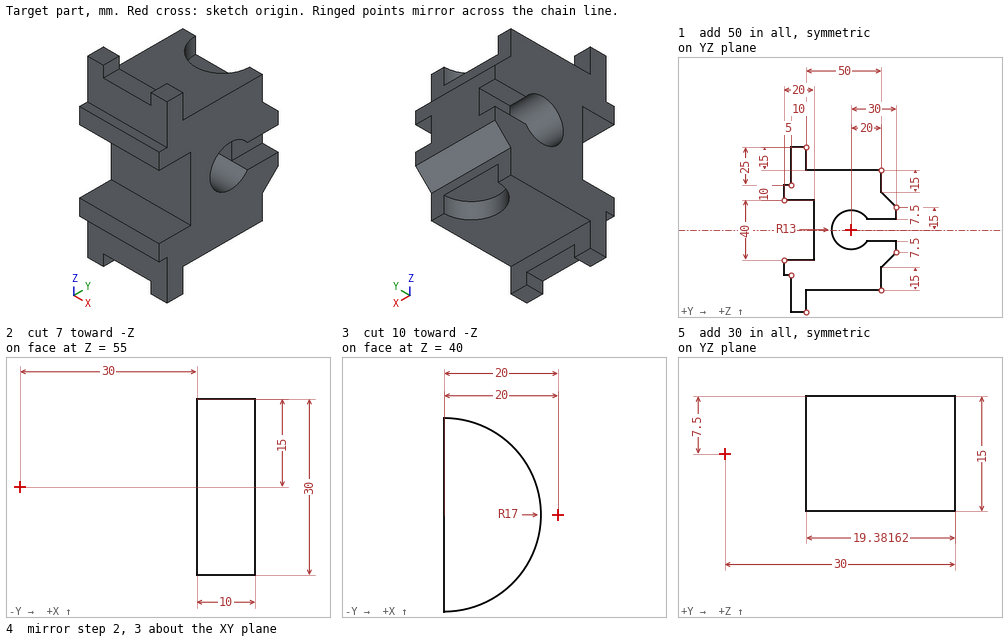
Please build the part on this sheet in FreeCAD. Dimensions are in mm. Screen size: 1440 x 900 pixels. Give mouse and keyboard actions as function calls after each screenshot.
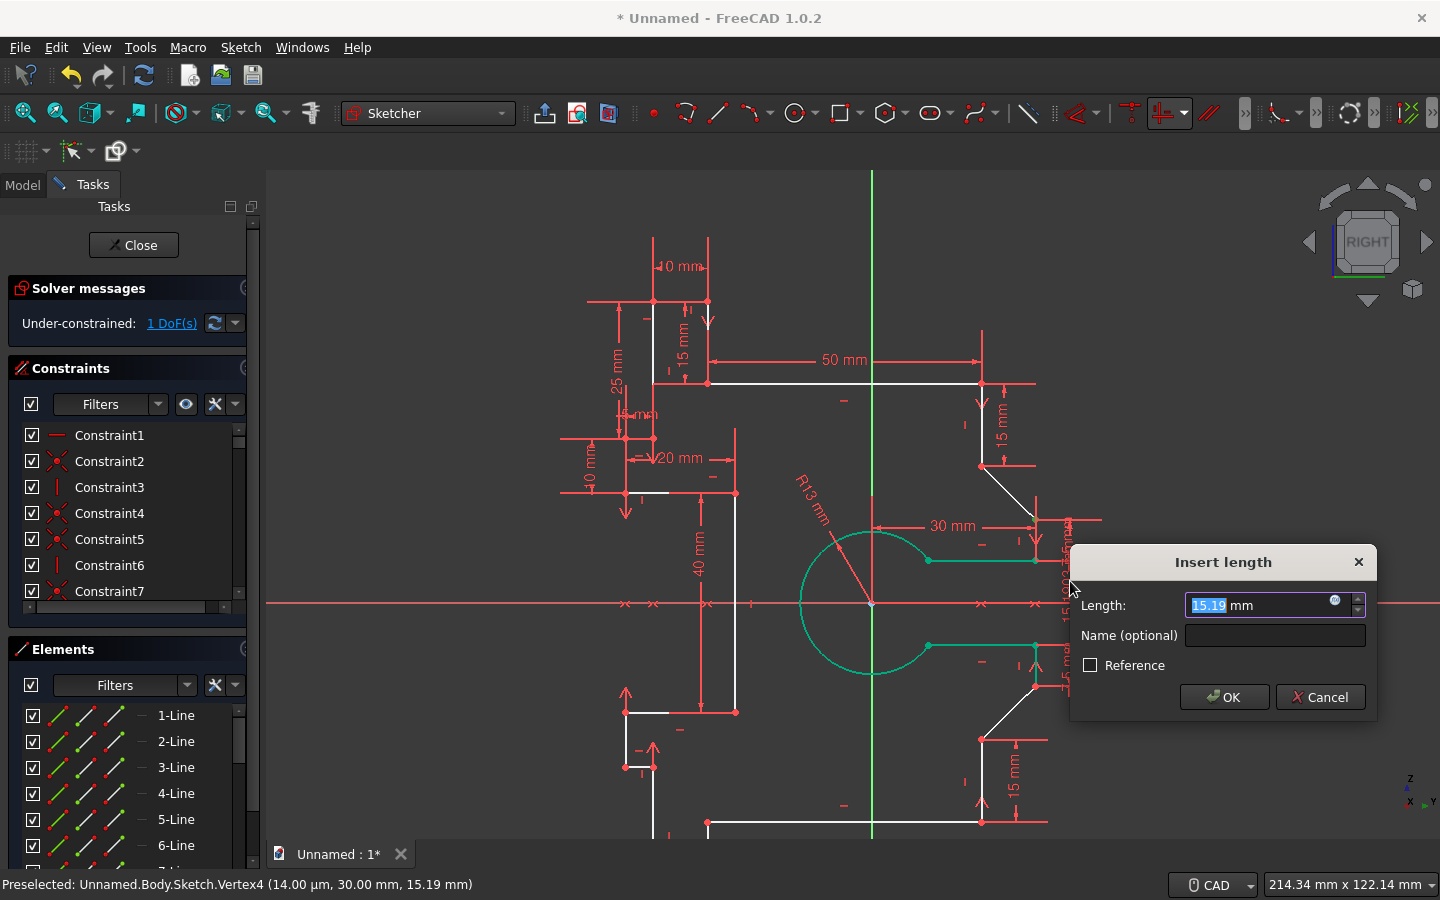
text(15)
key(Return)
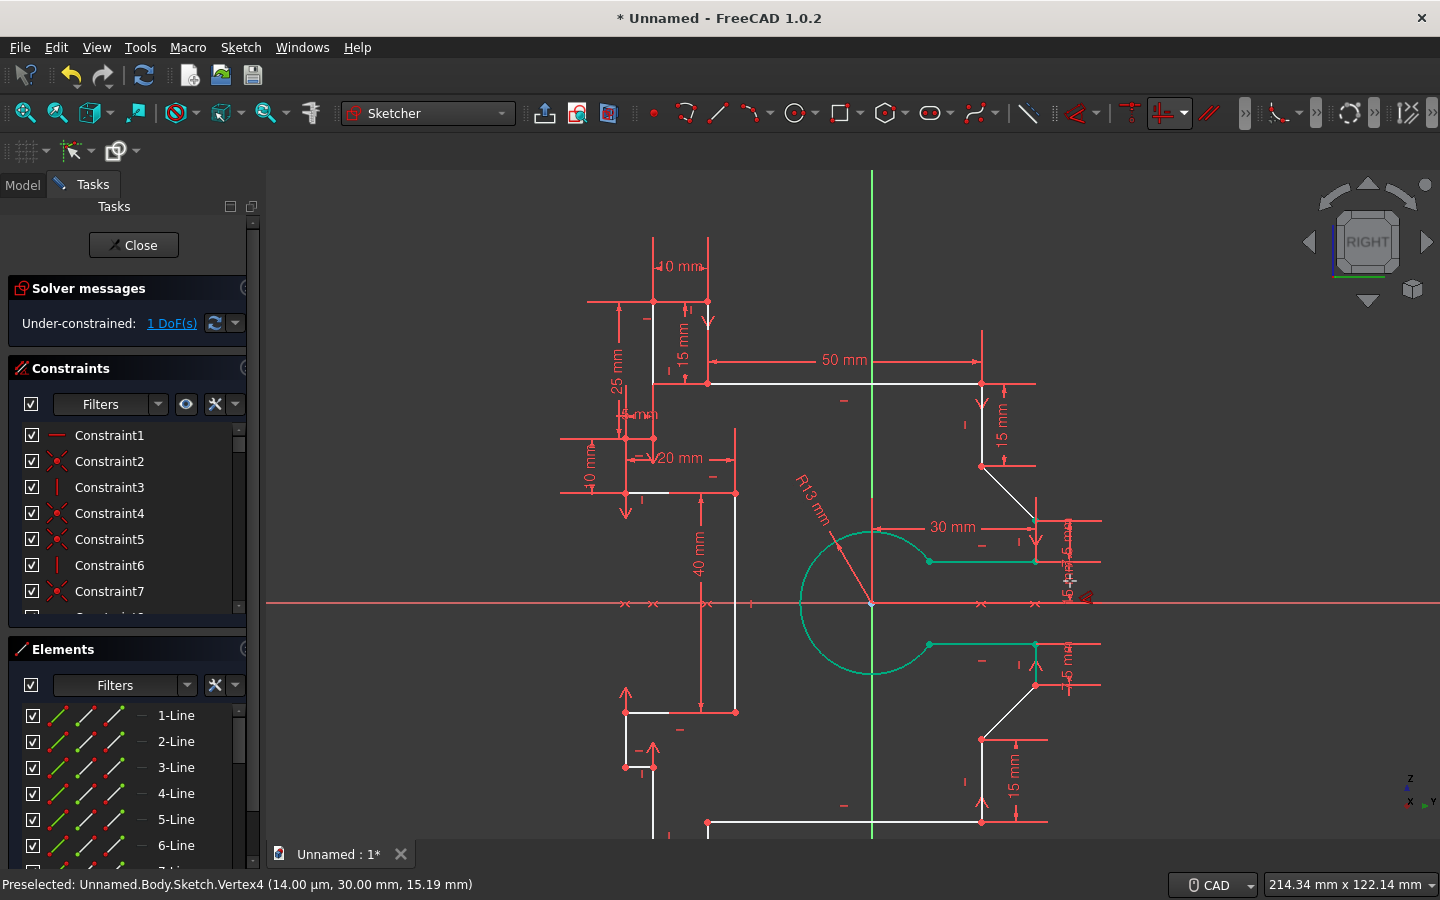
click(982, 466)
click(927, 432)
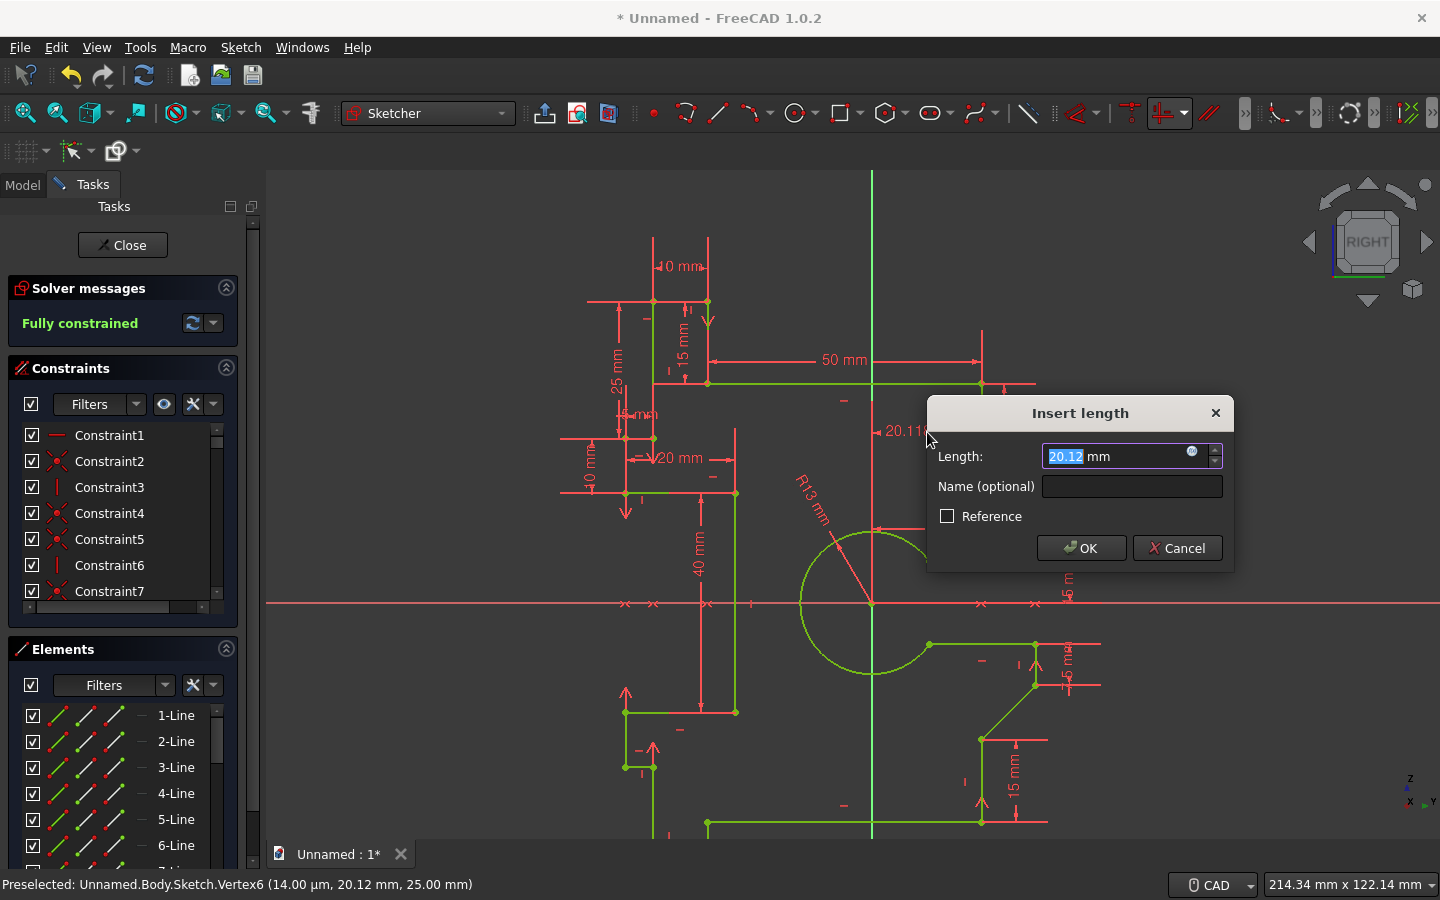
text(20)
key(Return)
key(Escape)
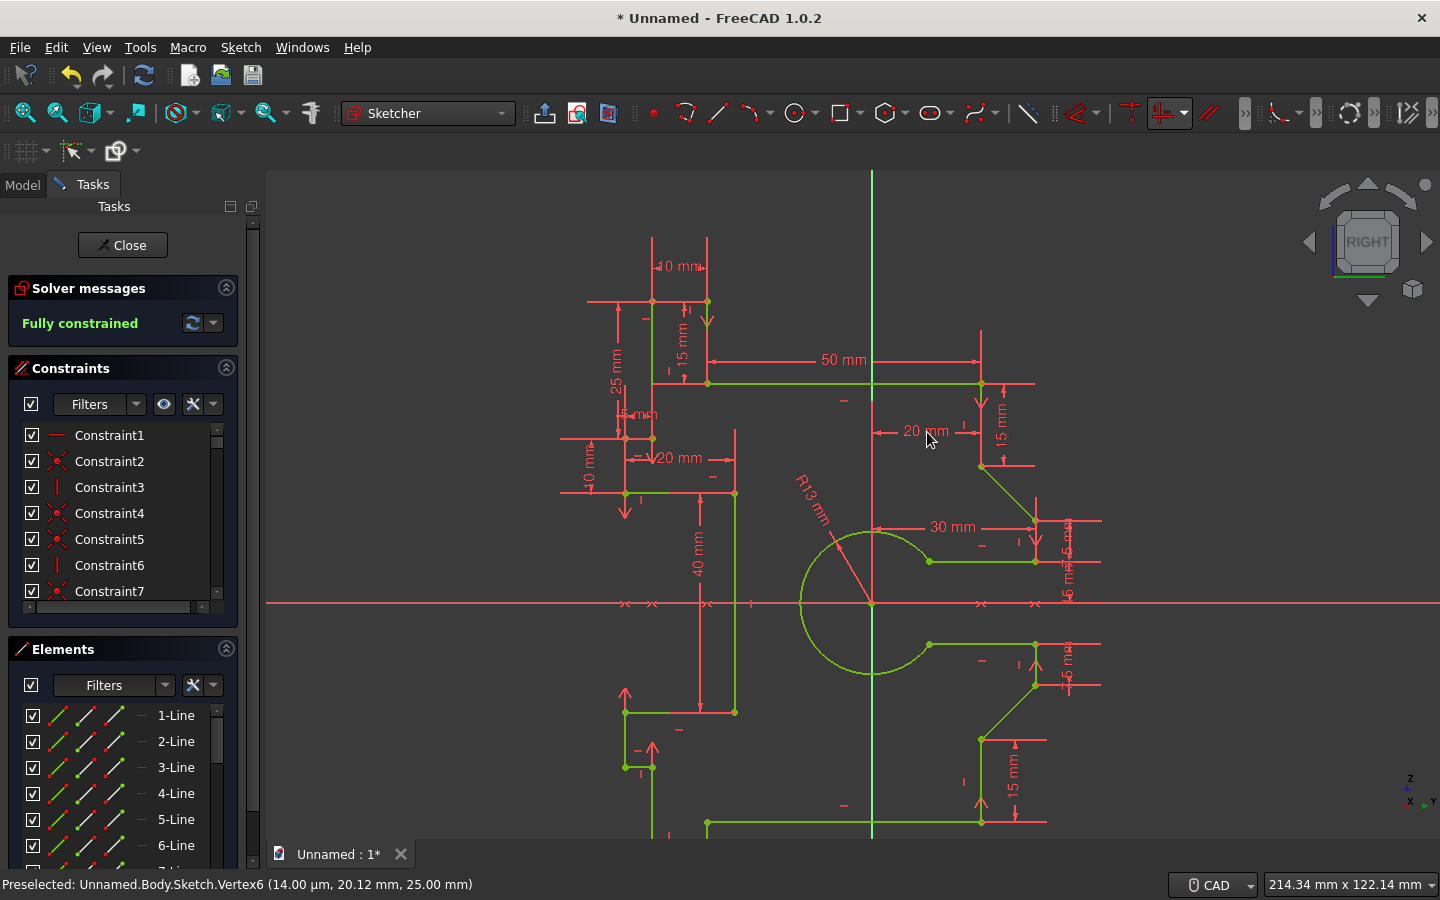
click(123, 245)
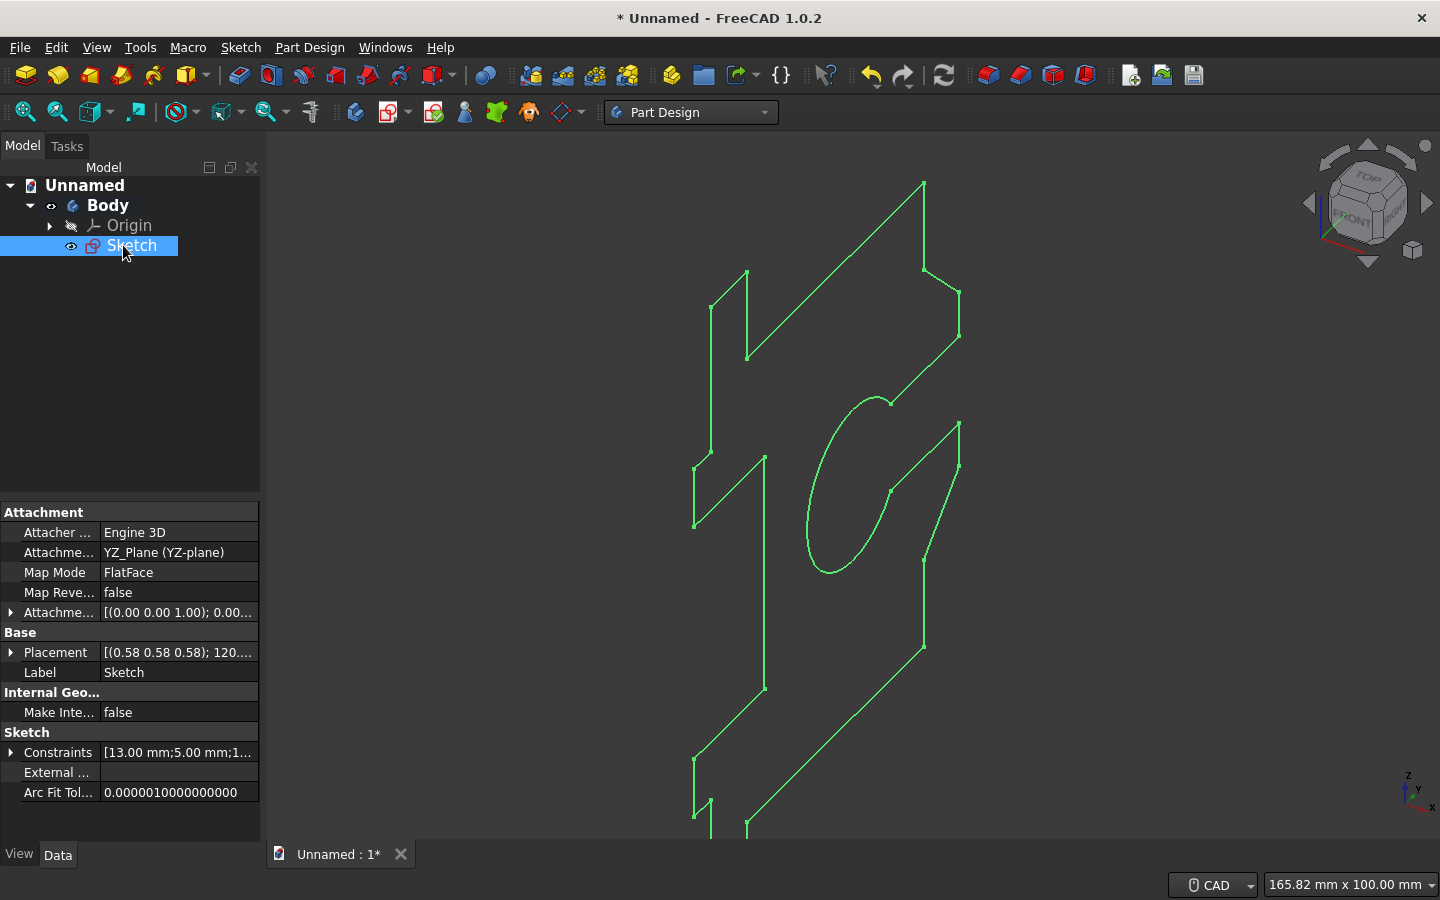
click(26, 76)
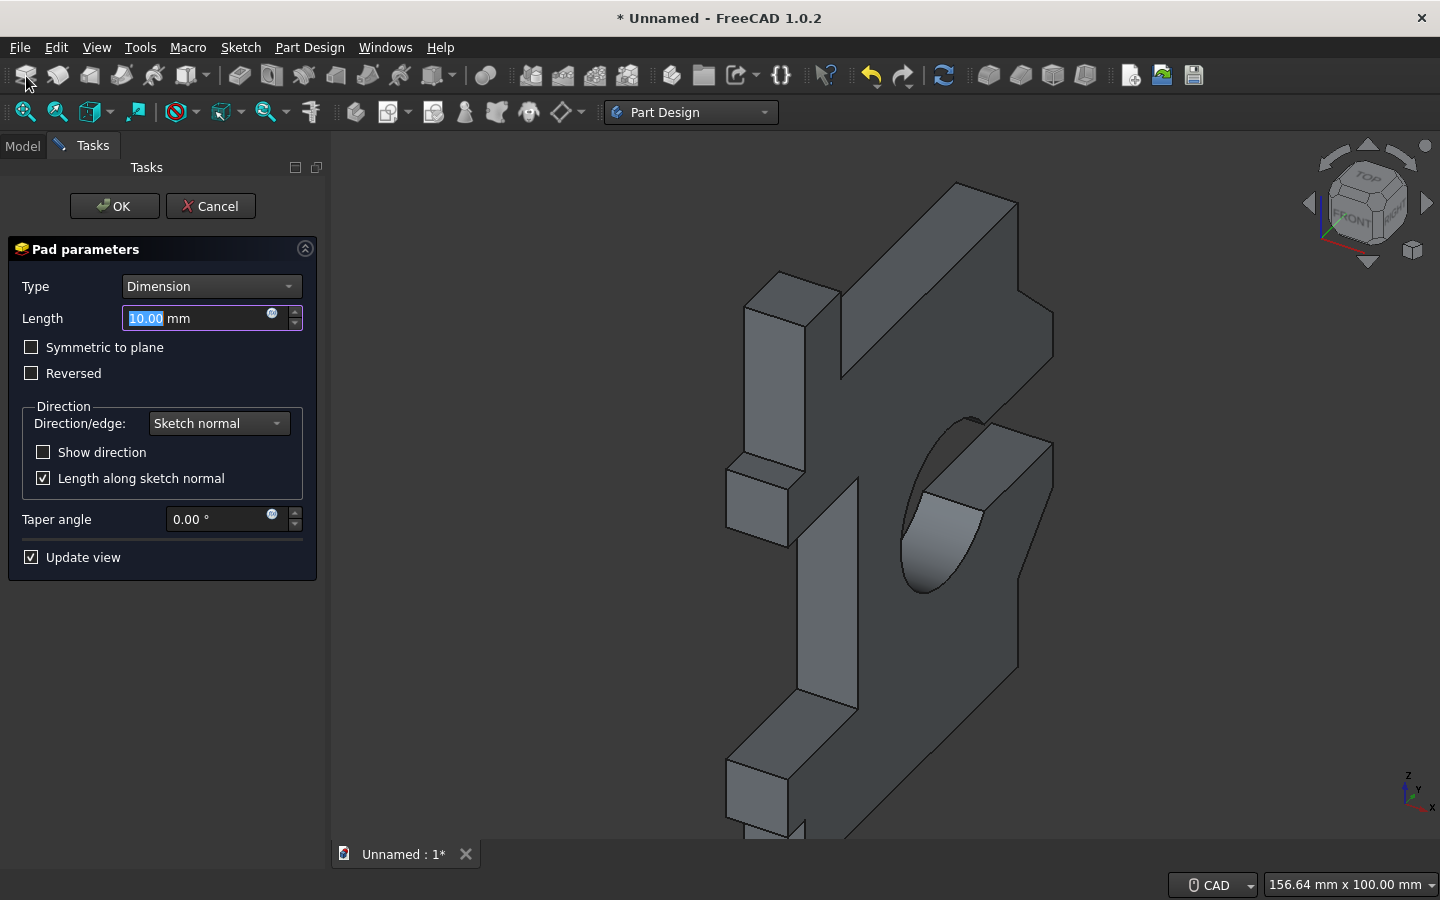
text(50)
key(Tab)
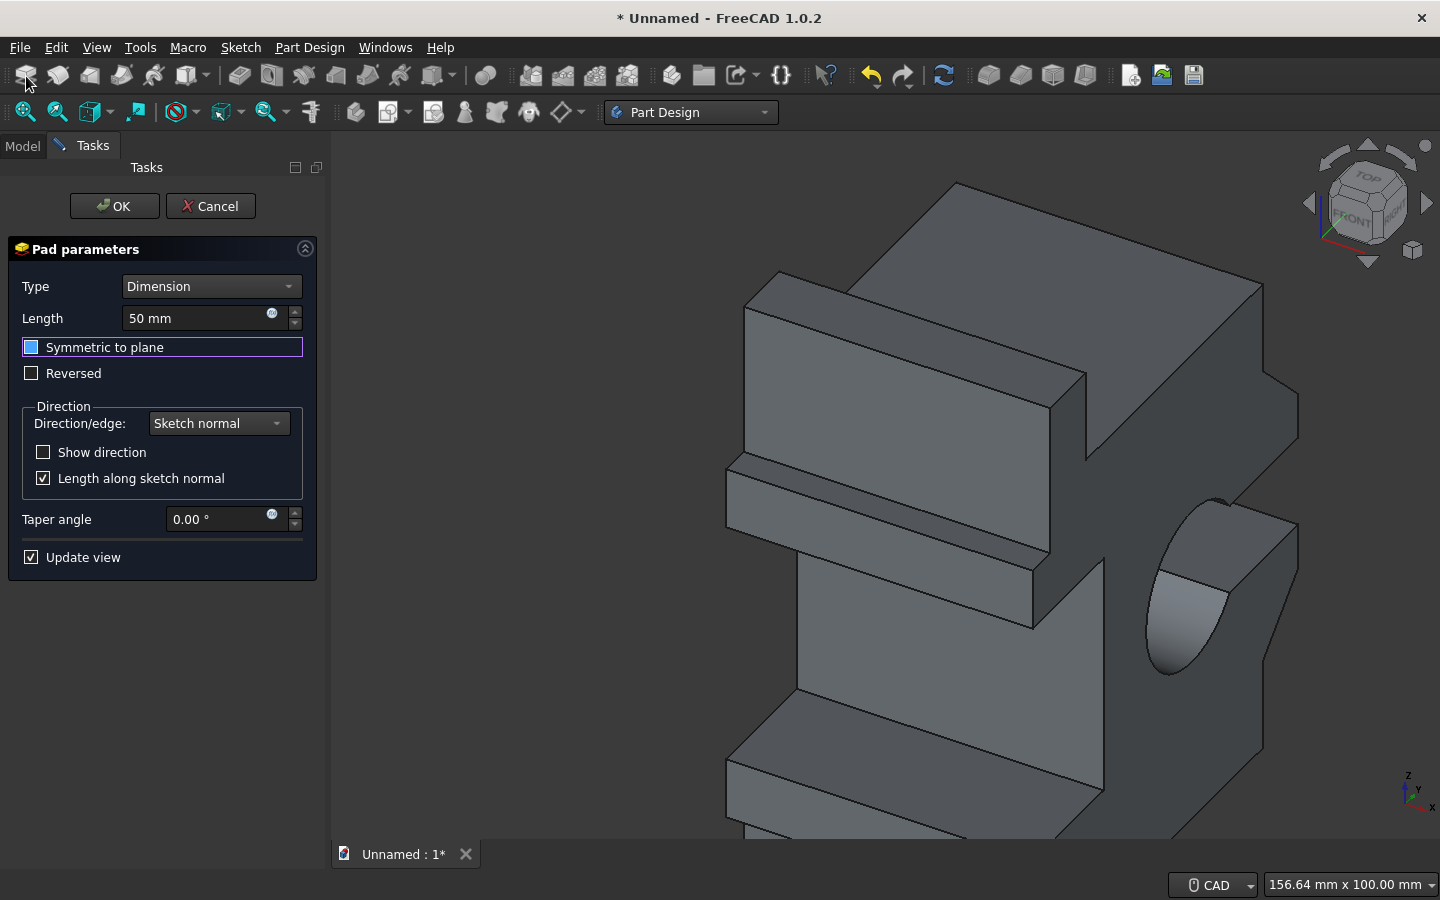
click(30, 347)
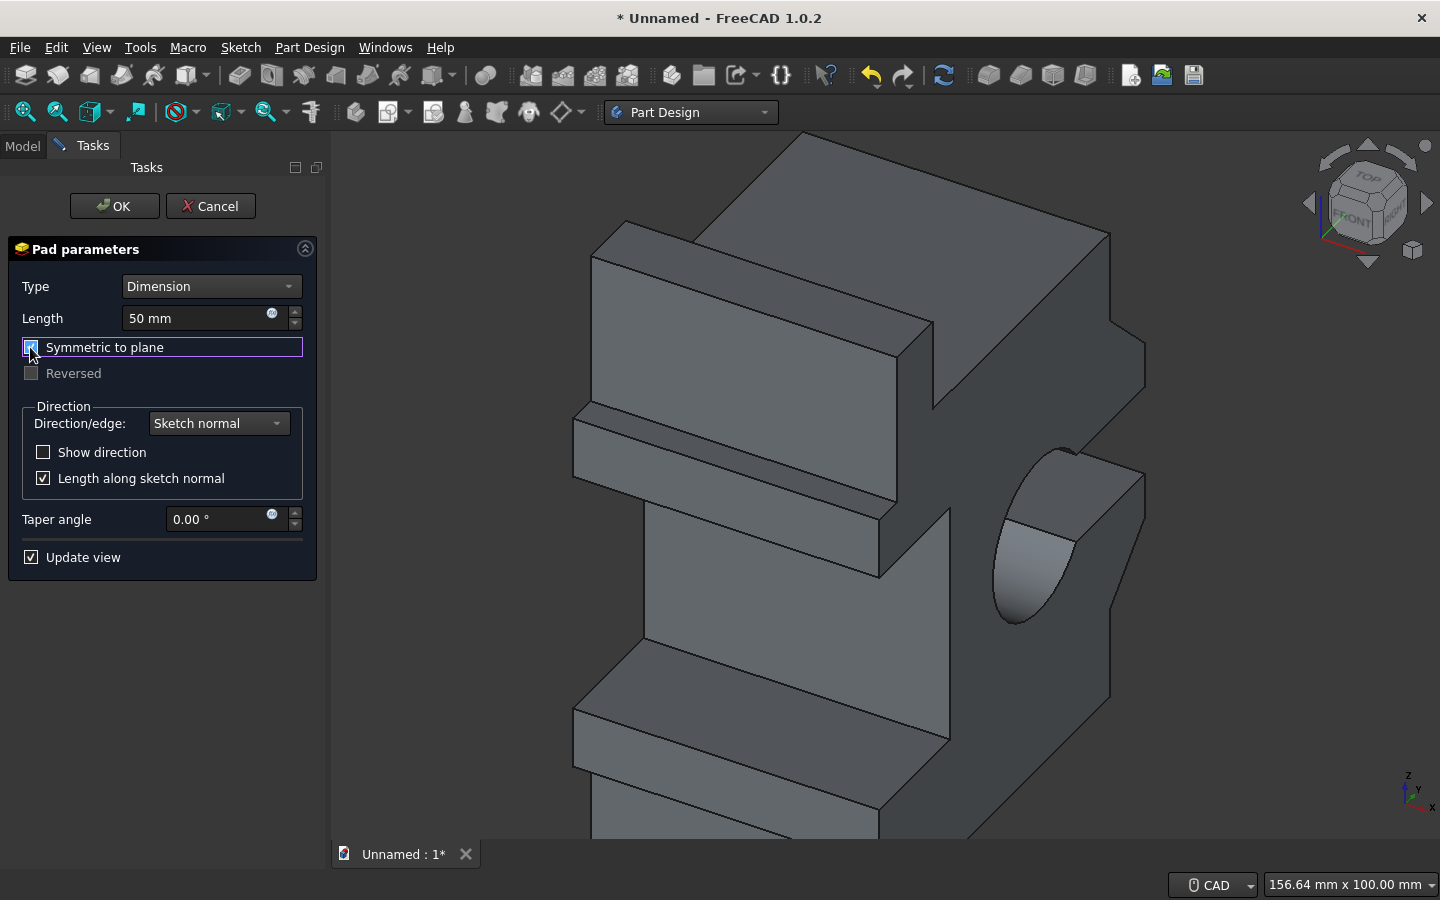
click(115, 206)